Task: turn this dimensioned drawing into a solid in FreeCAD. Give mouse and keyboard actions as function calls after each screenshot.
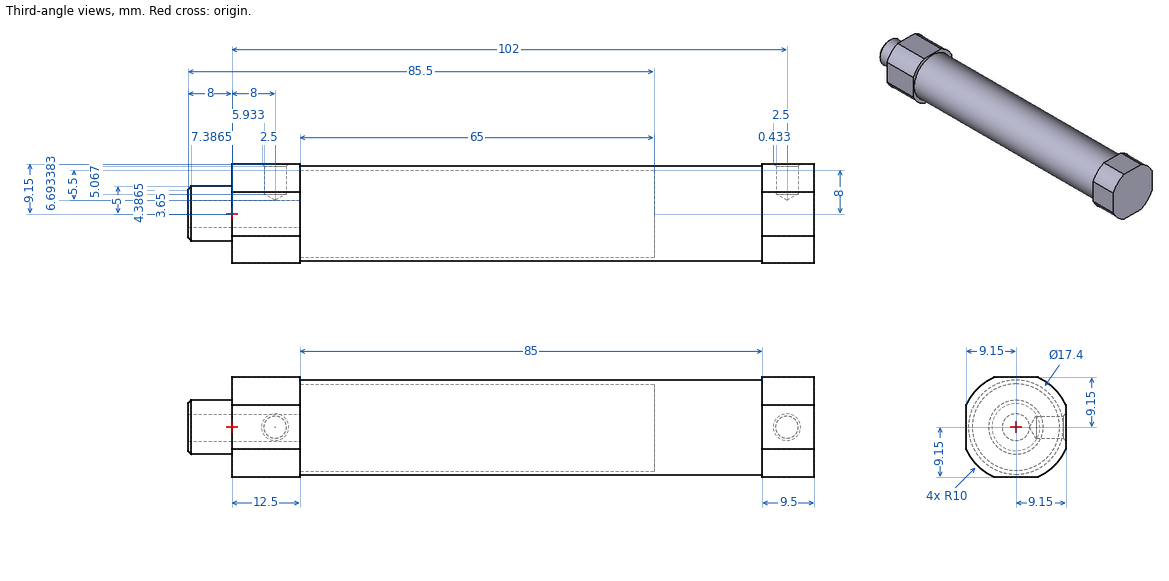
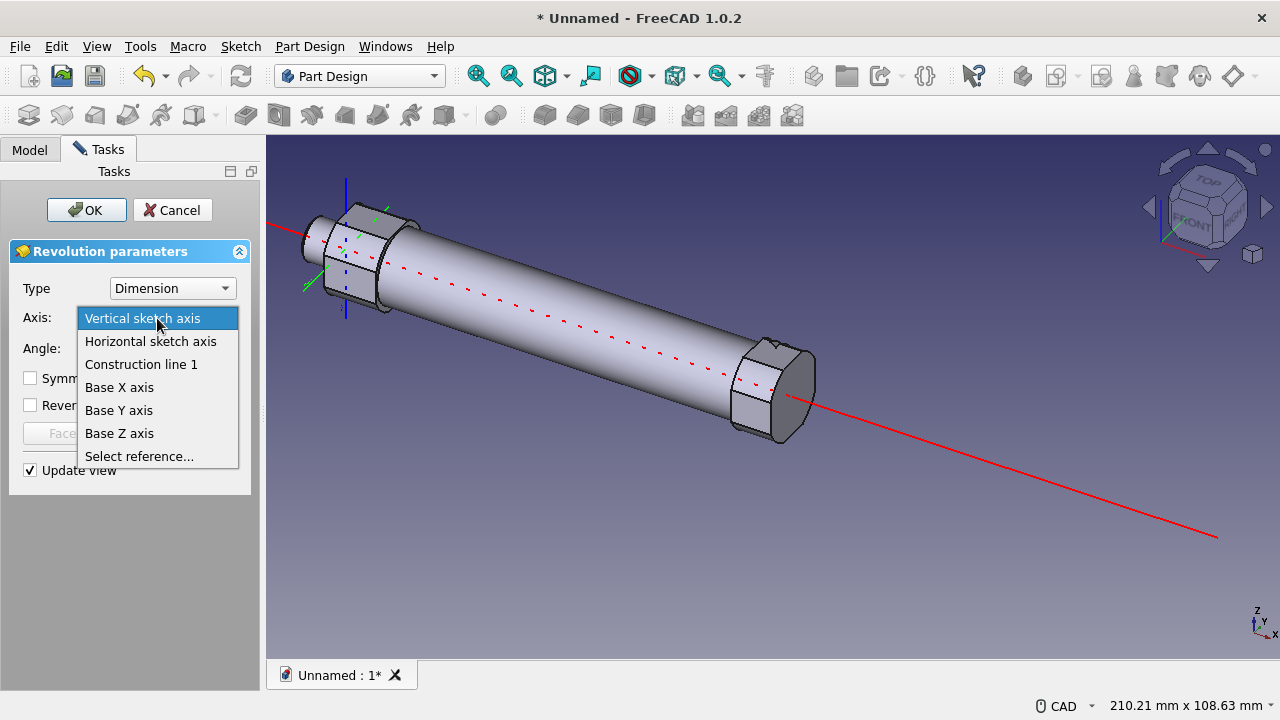
click(156, 364)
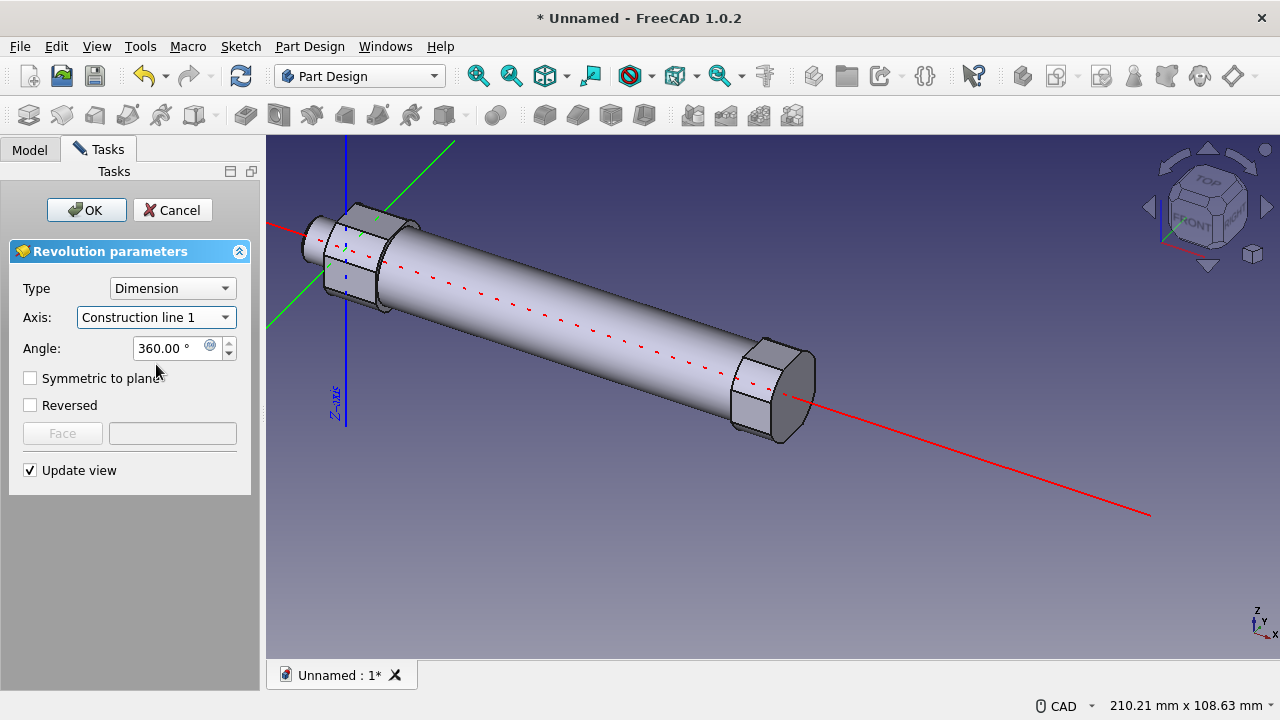
click(87, 210)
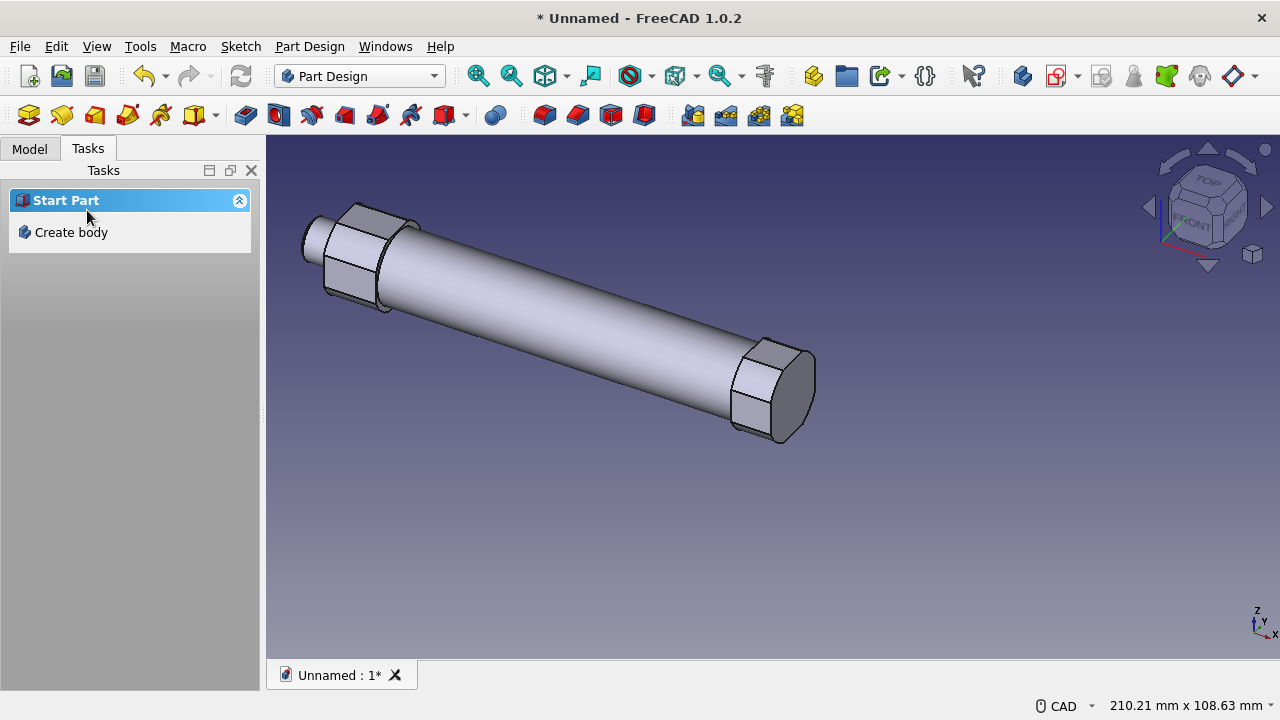
click(1056, 76)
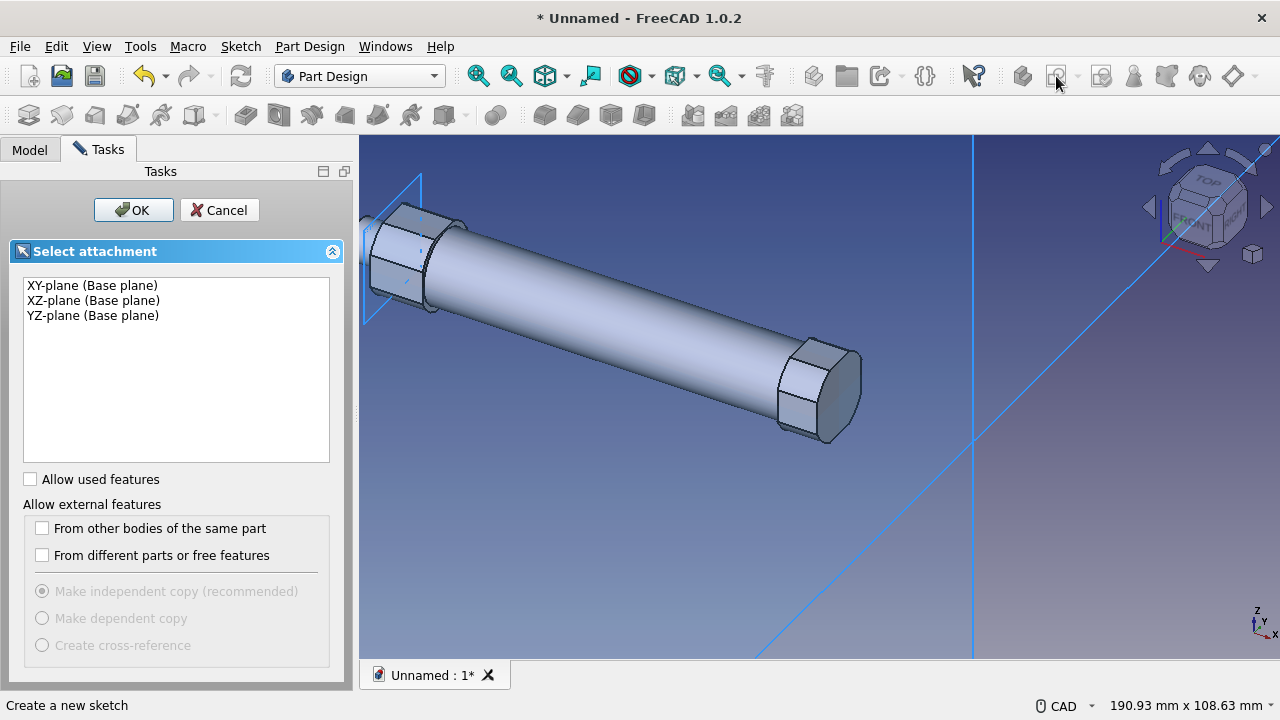
click(84, 286)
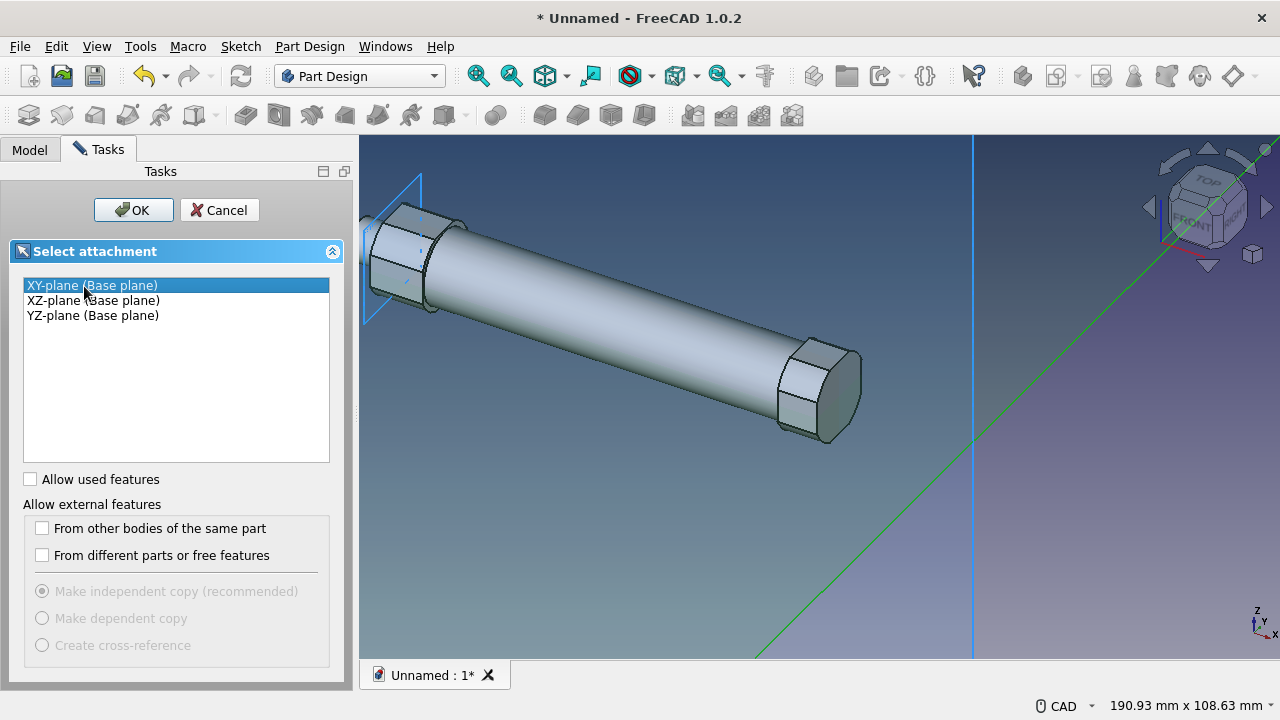
click(134, 210)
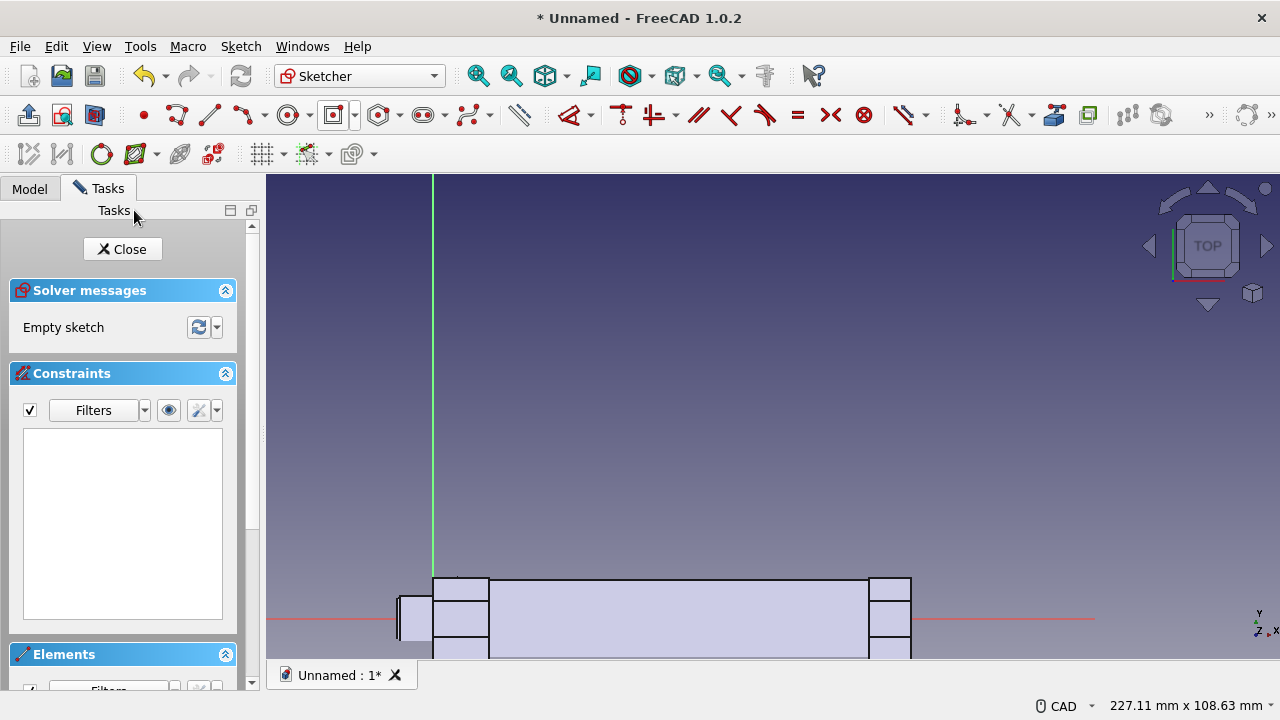
click(95, 116)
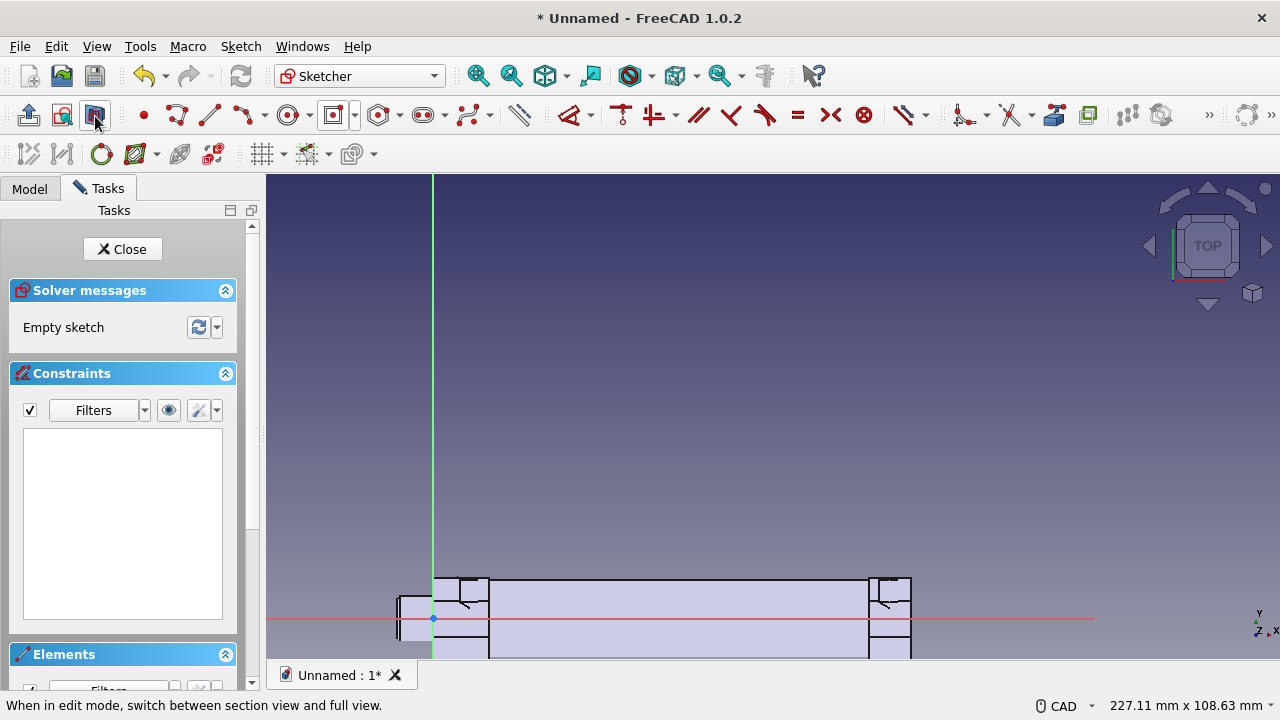
scroll(1115, 202, down, 1)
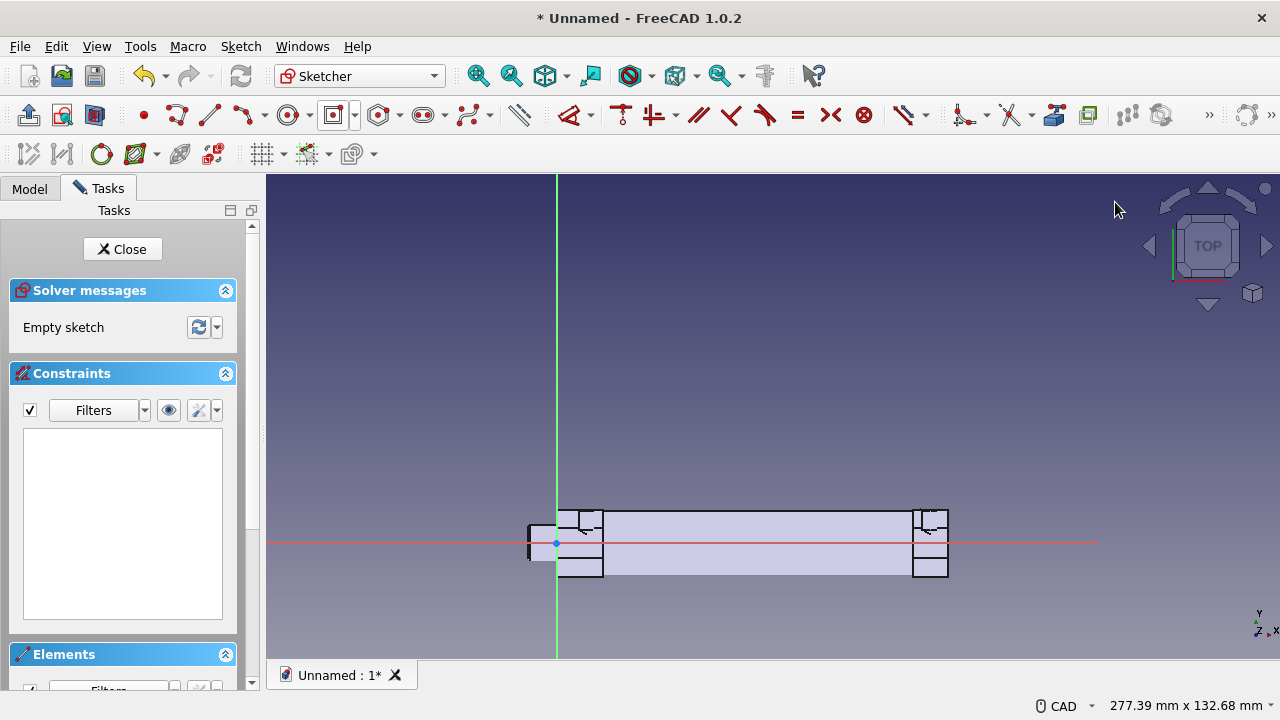
scroll(659, 631, up, 3)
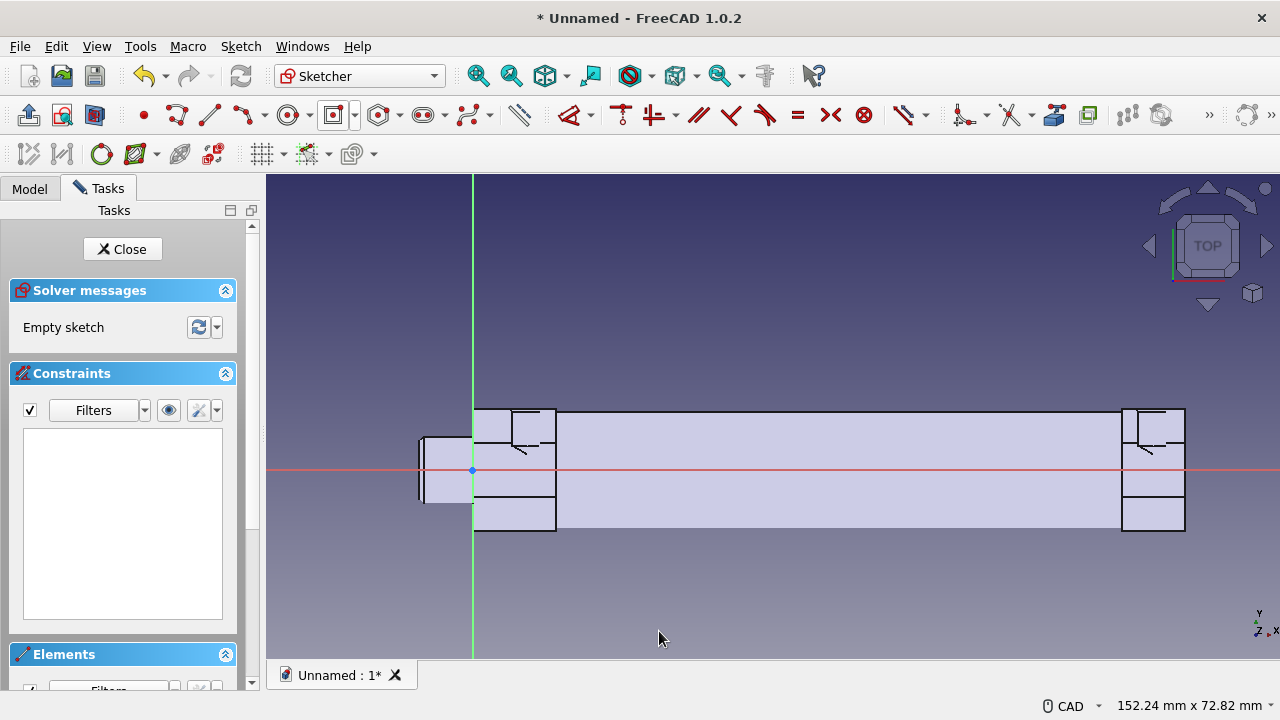
click(177, 116)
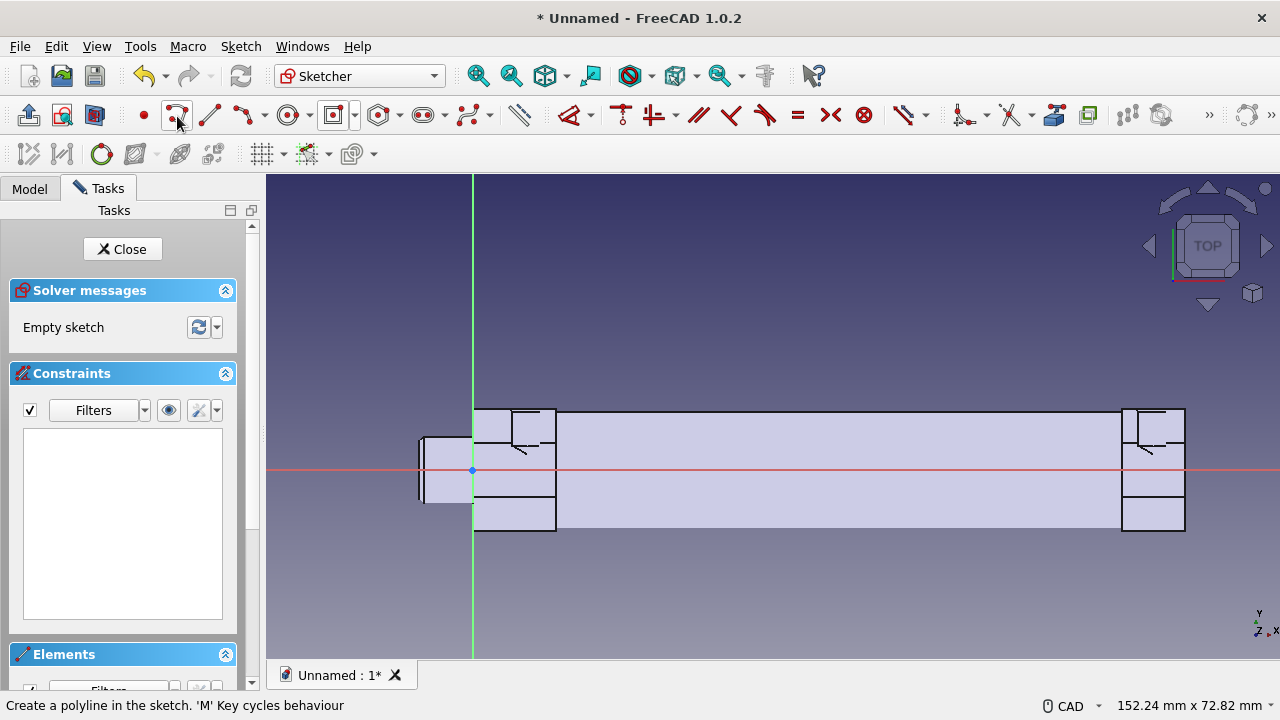
click(419, 470)
click(989, 461)
click(989, 417)
click(556, 417)
click(556, 453)
click(419, 453)
click(419, 470)
key(Escape)
key(Escape)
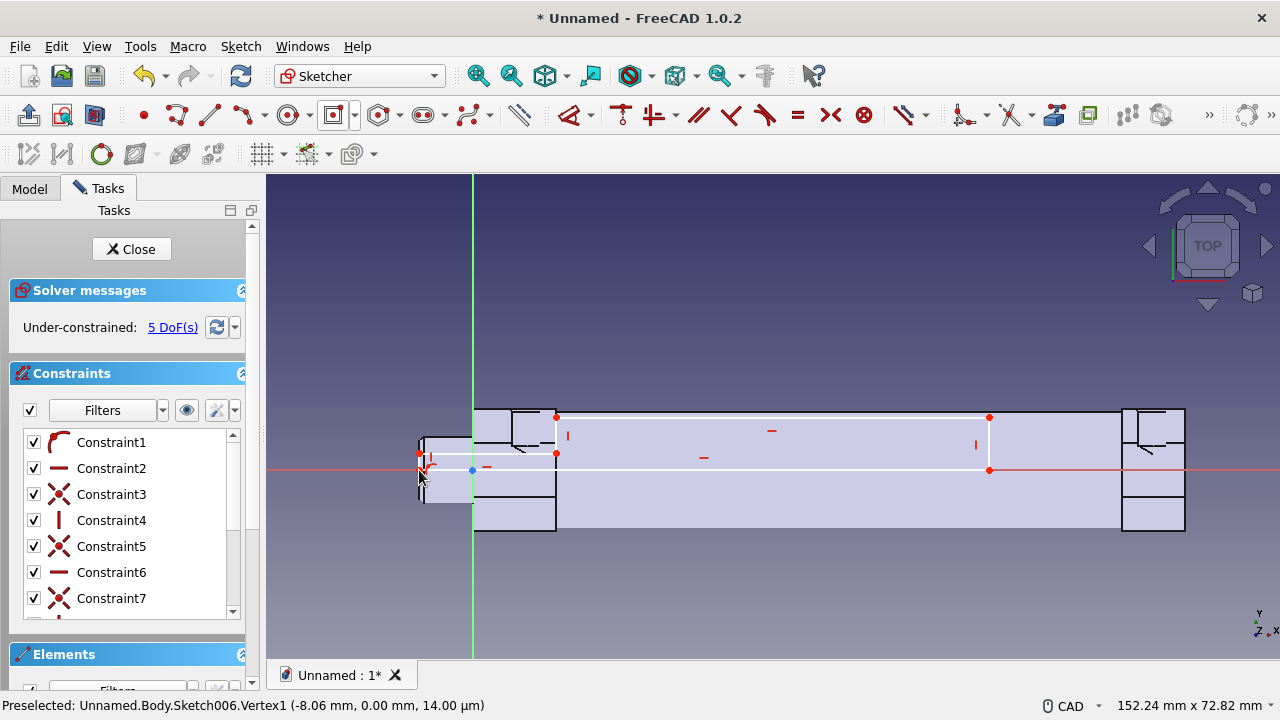
click(568, 116)